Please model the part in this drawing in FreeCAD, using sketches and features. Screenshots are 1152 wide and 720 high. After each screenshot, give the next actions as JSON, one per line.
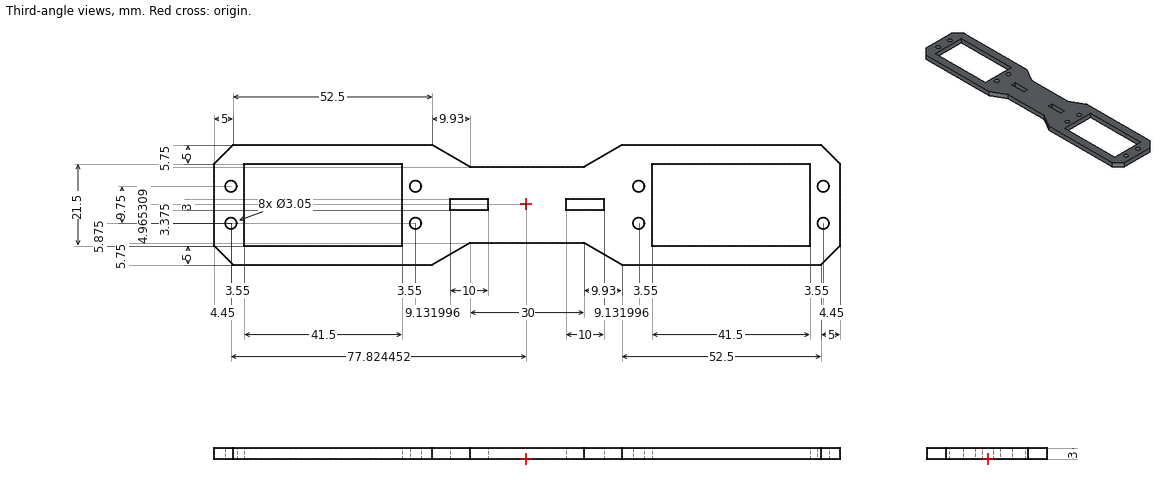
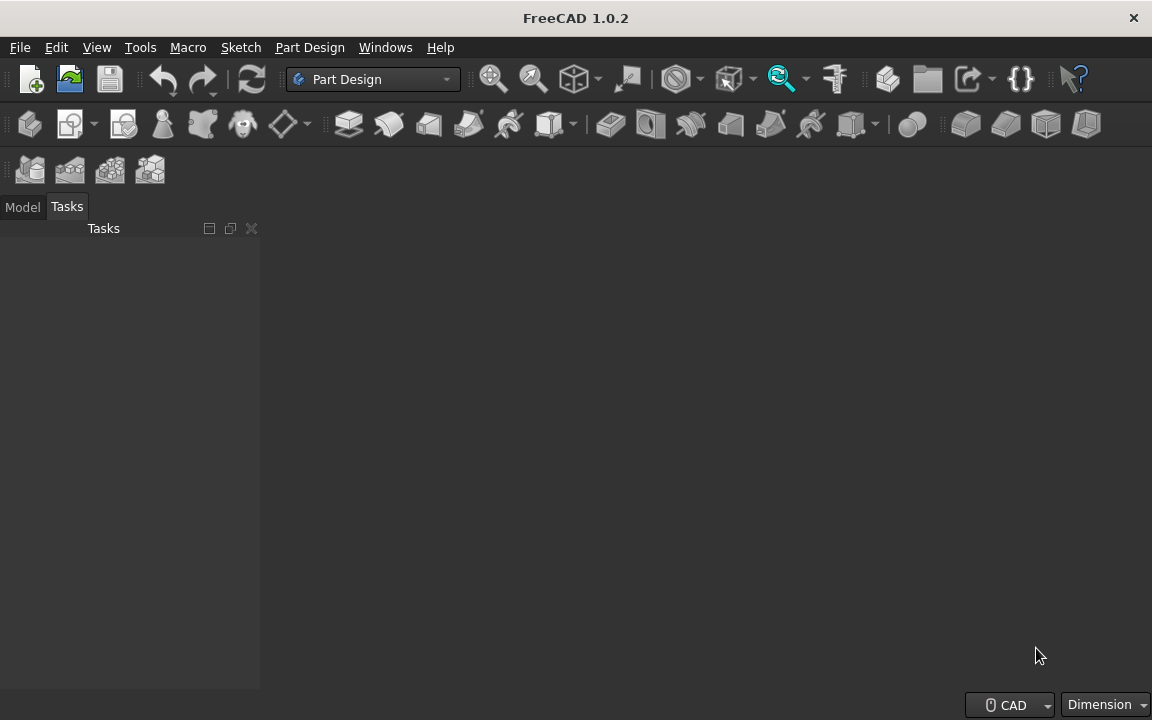
{"action": "left_click", "coordinate": [30, 80]}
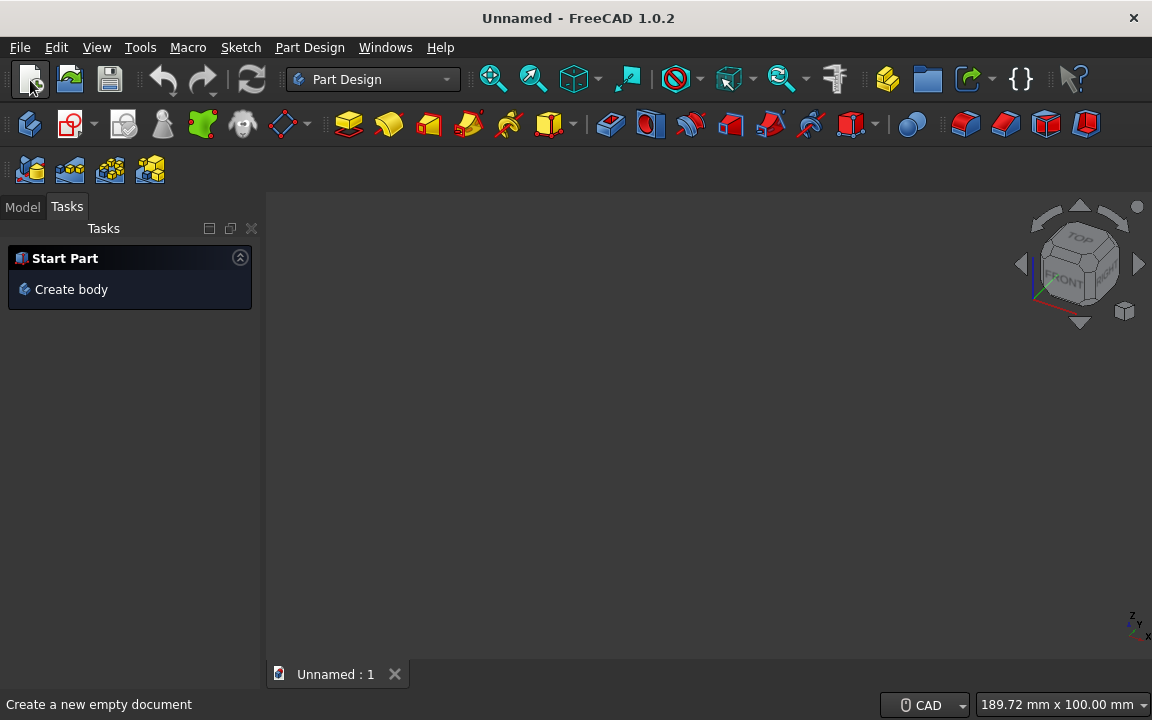
{"action": "left_click", "coordinate": [70, 124]}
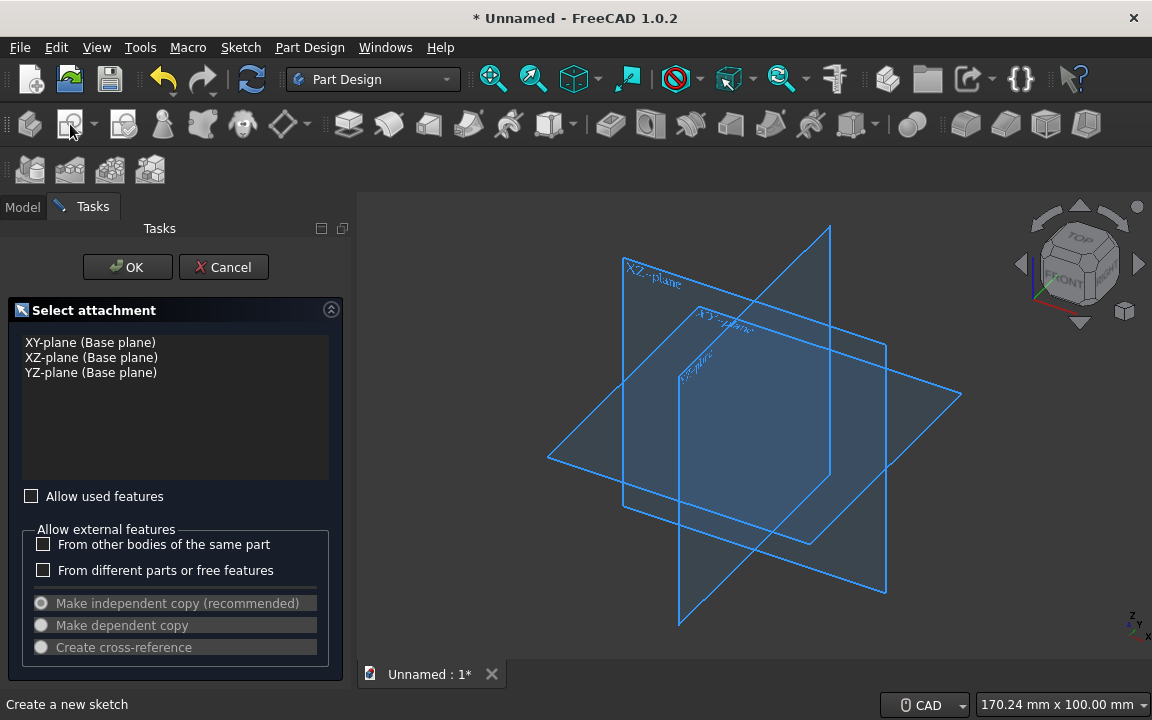
{"action": "left_click", "coordinate": [82, 342]}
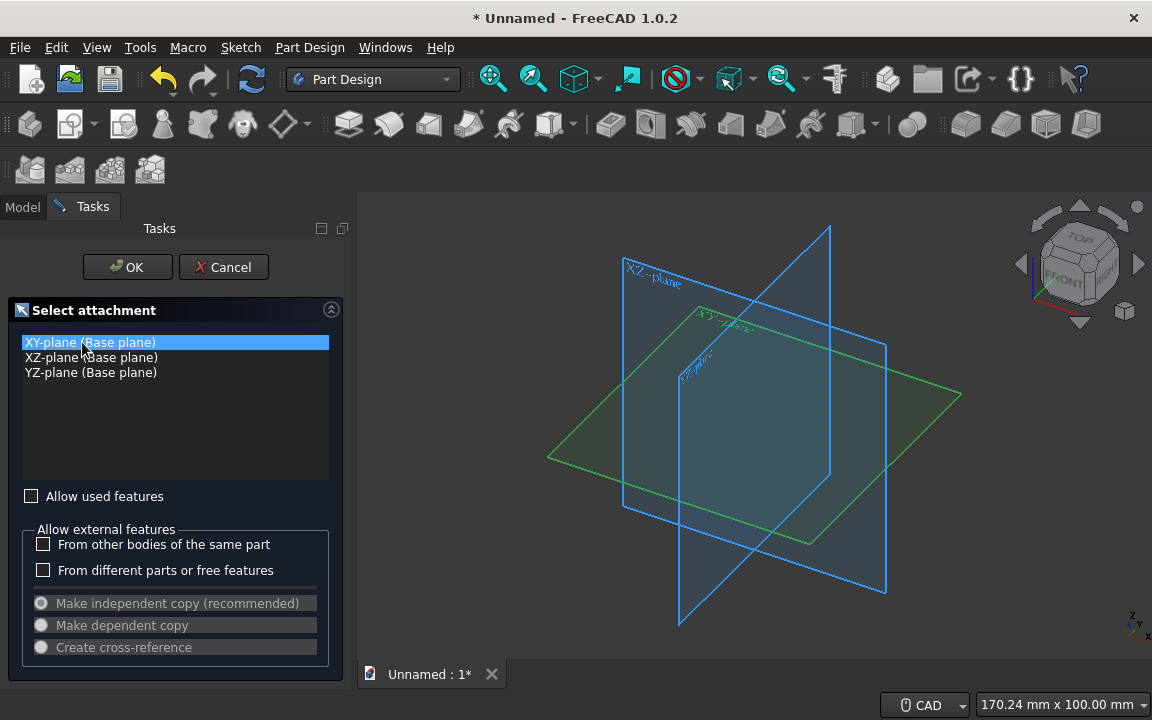
{"action": "left_click", "coordinate": [128, 267]}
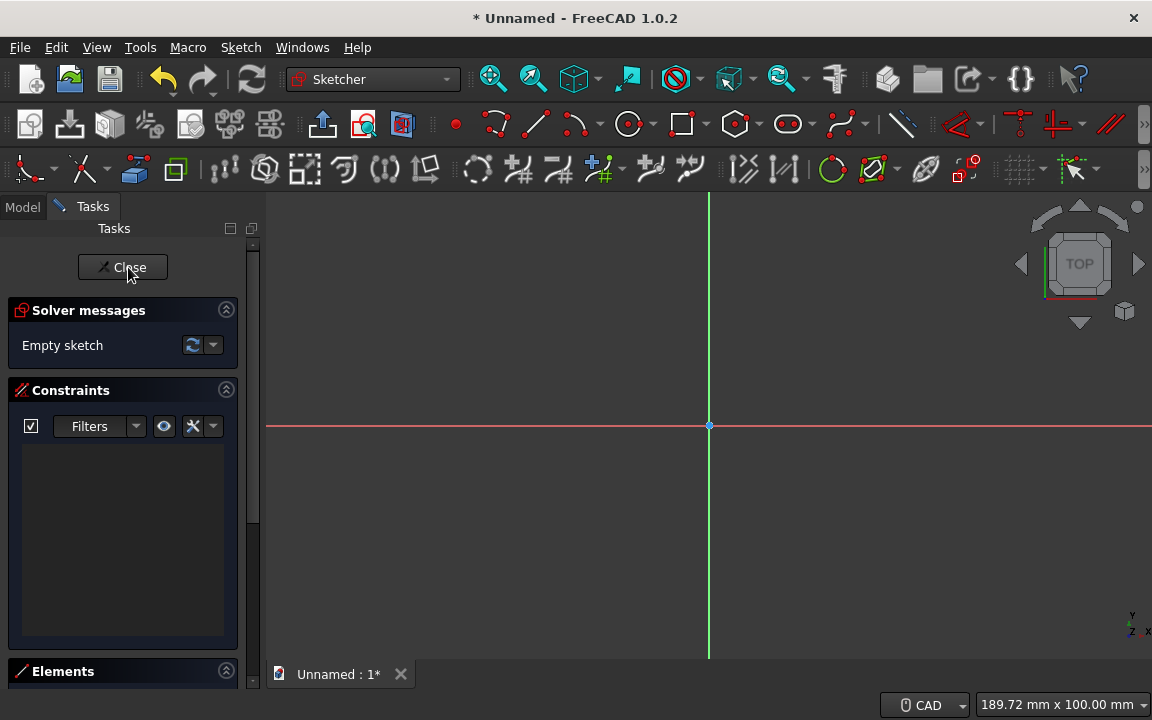
{"action": "scroll", "coordinate": [500, 425], "scroll_direction": "down", "scroll_amount": 2}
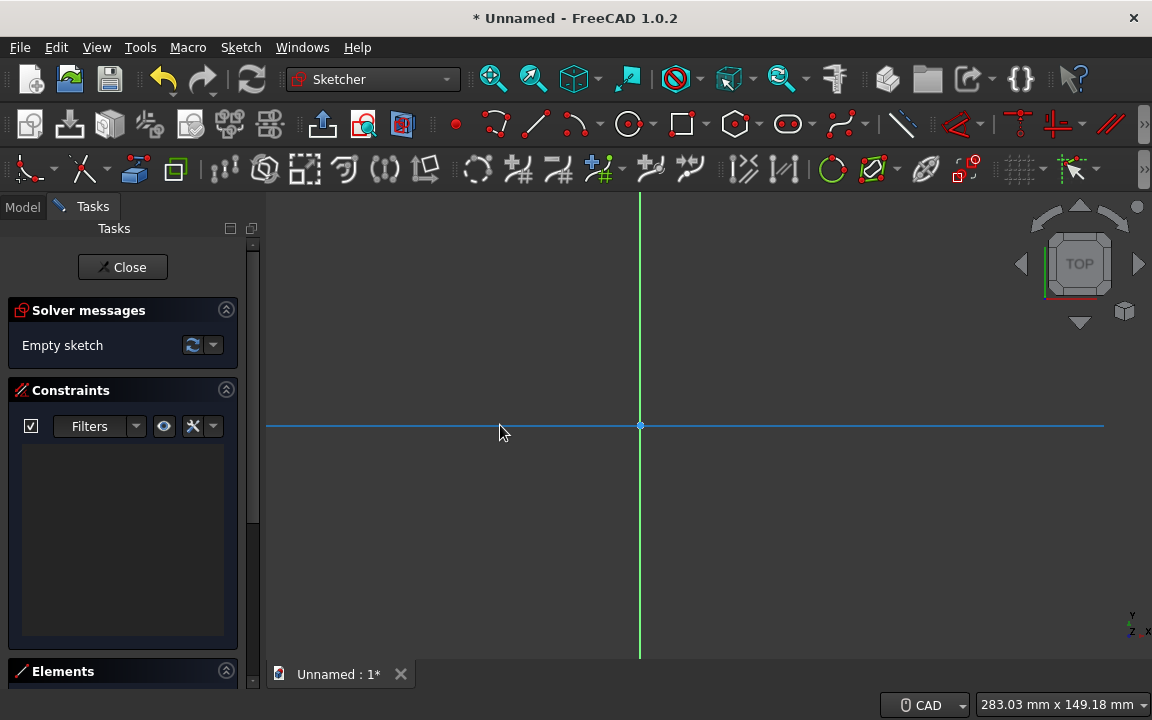
{"action": "left_click", "coordinate": [496, 124]}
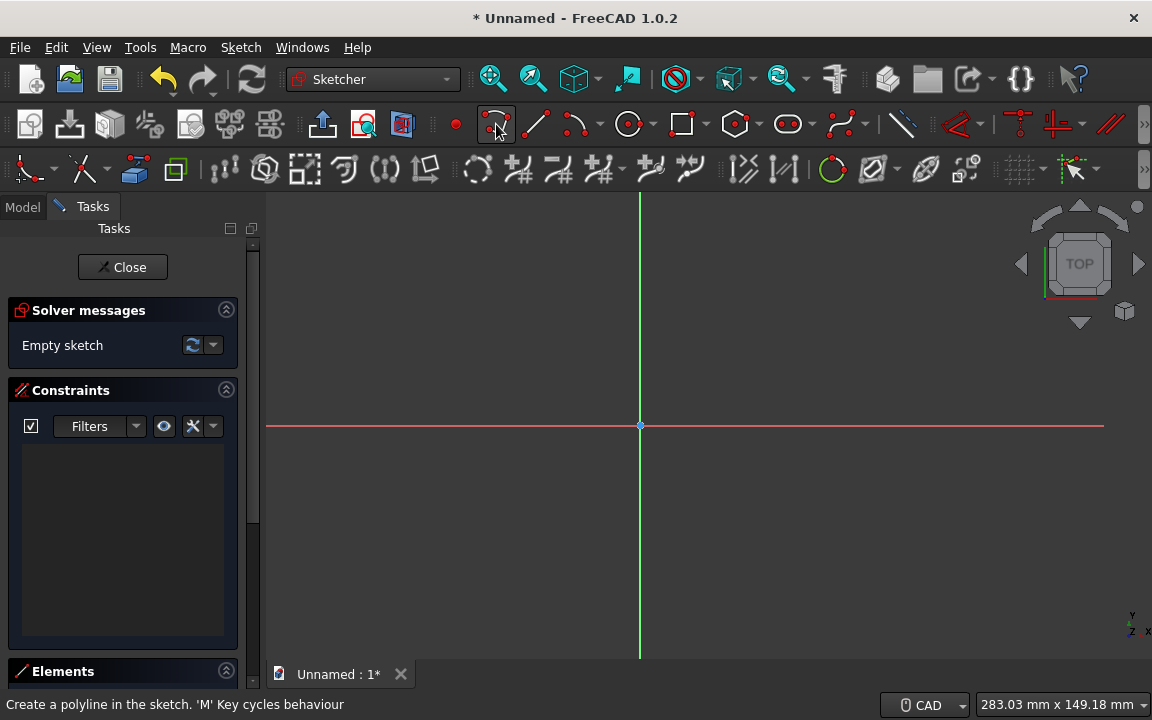
{"action": "left_click", "coordinate": [594, 394]}
{"action": "left_click", "coordinate": [563, 376]}
{"action": "left_click", "coordinate": [398, 376]}
{"action": "left_click", "coordinate": [383, 392]}
{"action": "left_click", "coordinate": [383, 459]}
{"action": "left_click", "coordinate": [398, 475]}
{"action": "left_click", "coordinate": [563, 475]}
{"action": "left_click", "coordinate": [594, 457]}
{"action": "left_click", "coordinate": [688, 457]}
{"action": "left_click", "coordinate": [719, 475]}
{"action": "left_click", "coordinate": [883, 475]}
{"action": "left_click", "coordinate": [899, 459]}
{"action": "left_click", "coordinate": [899, 392]}
{"action": "left_click", "coordinate": [883, 376]}
{"action": "left_click", "coordinate": [719, 376]}
{"action": "left_click", "coordinate": [688, 394]}
{"action": "left_click", "coordinate": [594, 395]}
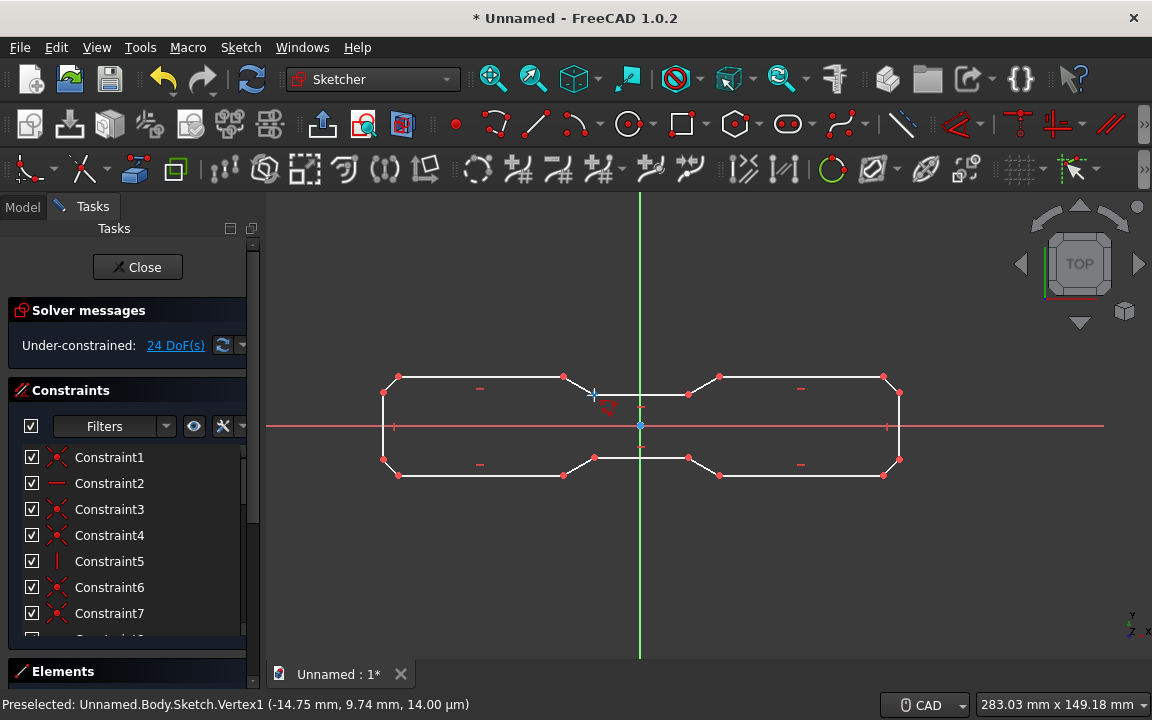
{"action": "left_click", "coordinate": [682, 124]}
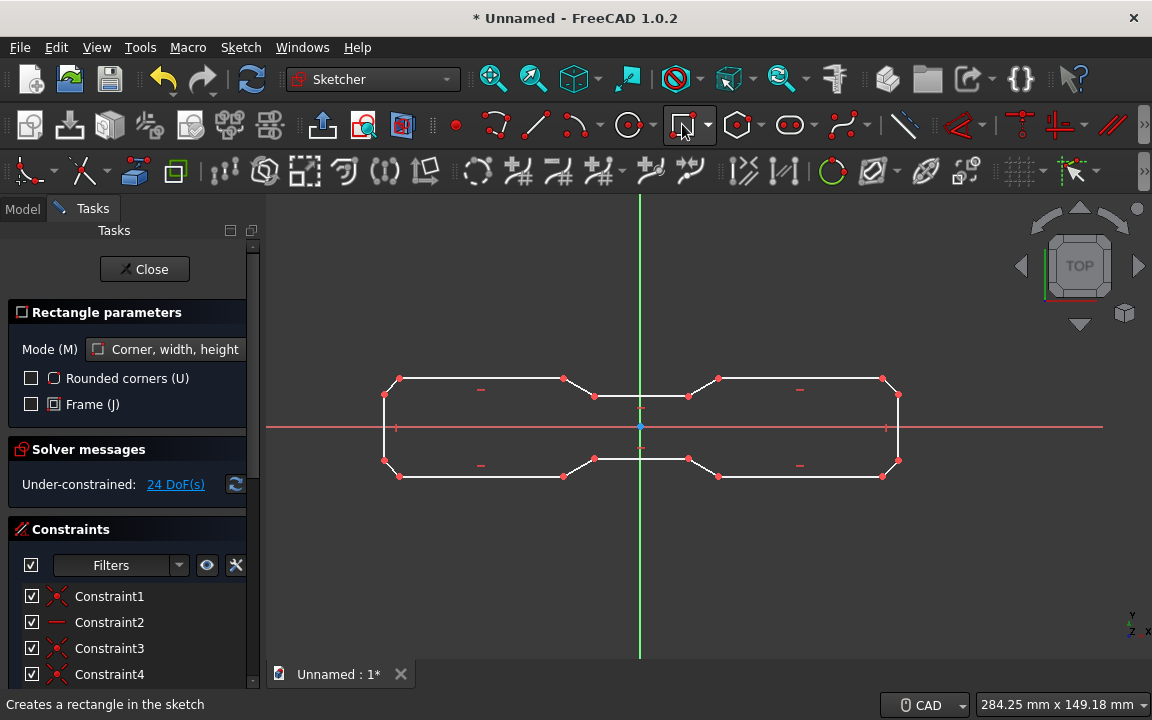
{"action": "left_click", "coordinate": [409, 393]}
{"action": "mouse_move", "coordinate": [538, 460]}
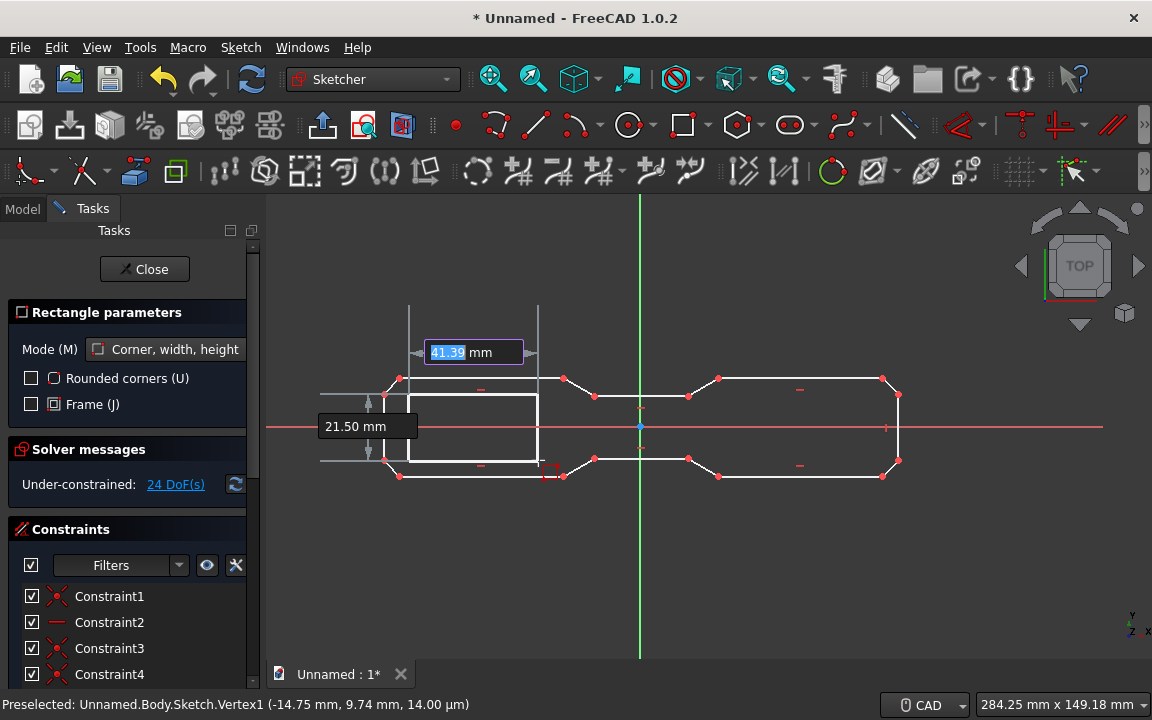
{"action": "type", "text": "41.5"}
{"action": "key", "text": "Tab"}
{"action": "type", "text": "21.5"}
{"action": "key", "text": "Return"}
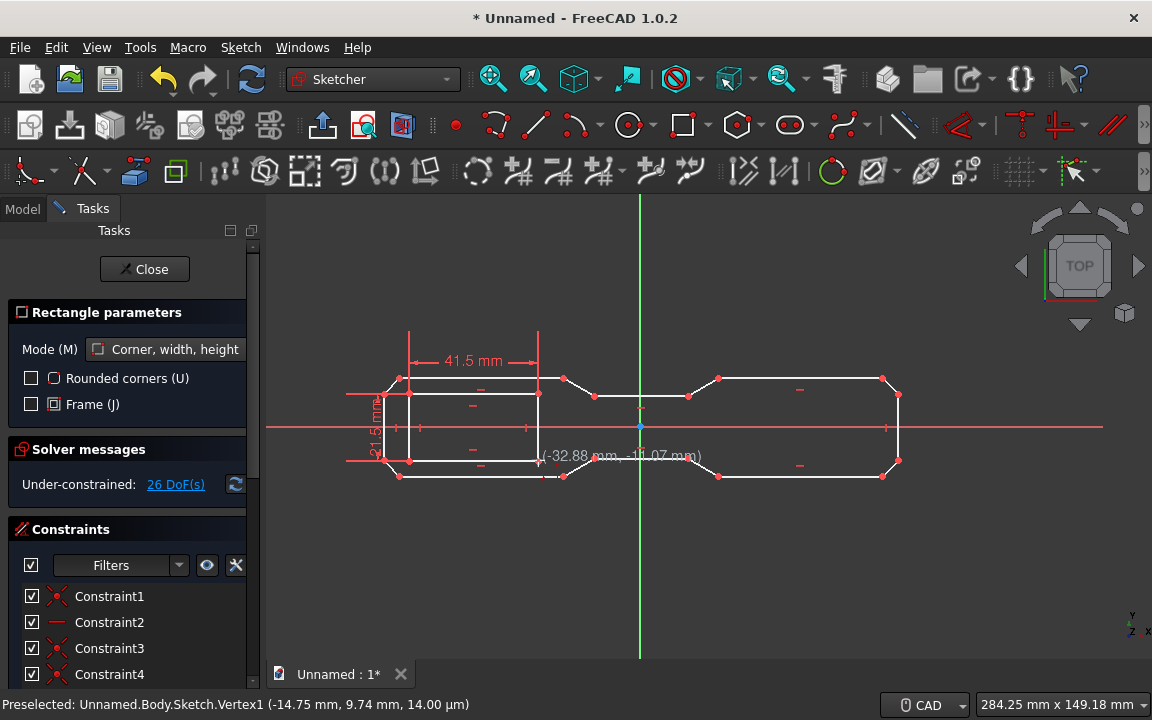
{"action": "scroll", "coordinate": [578, 422], "scroll_direction": "up", "scroll_amount": 7}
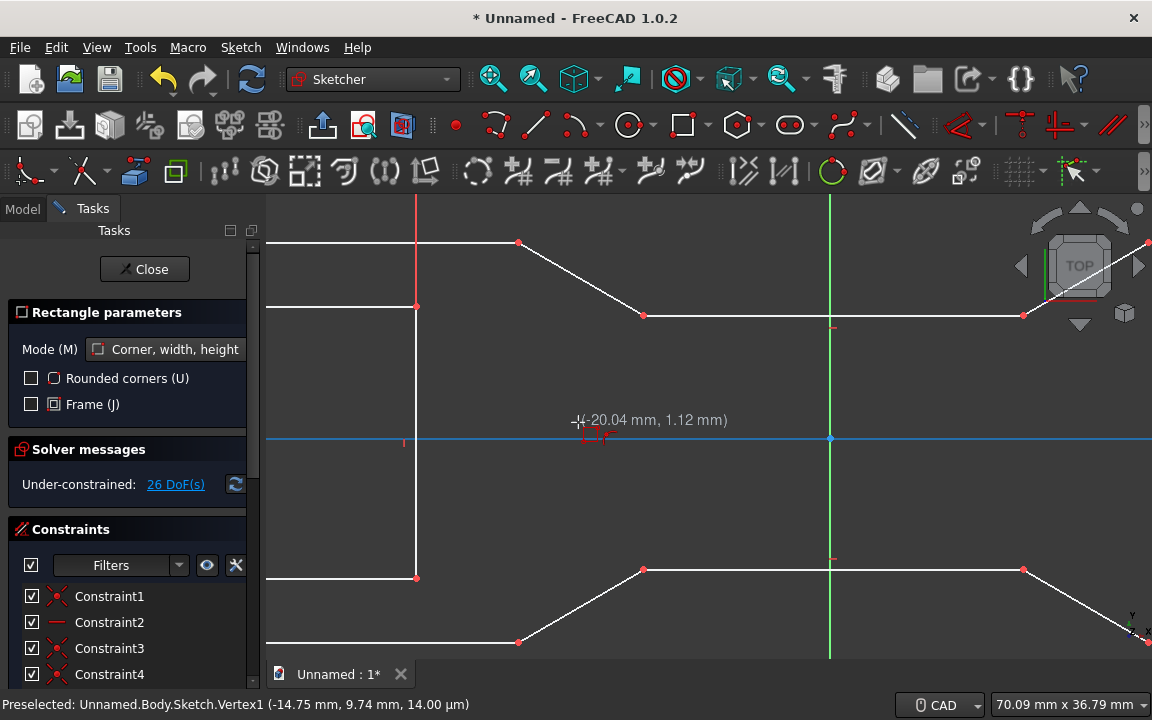
{"action": "left_click", "coordinate": [576, 421]}
{"action": "mouse_move", "coordinate": [703, 459]}